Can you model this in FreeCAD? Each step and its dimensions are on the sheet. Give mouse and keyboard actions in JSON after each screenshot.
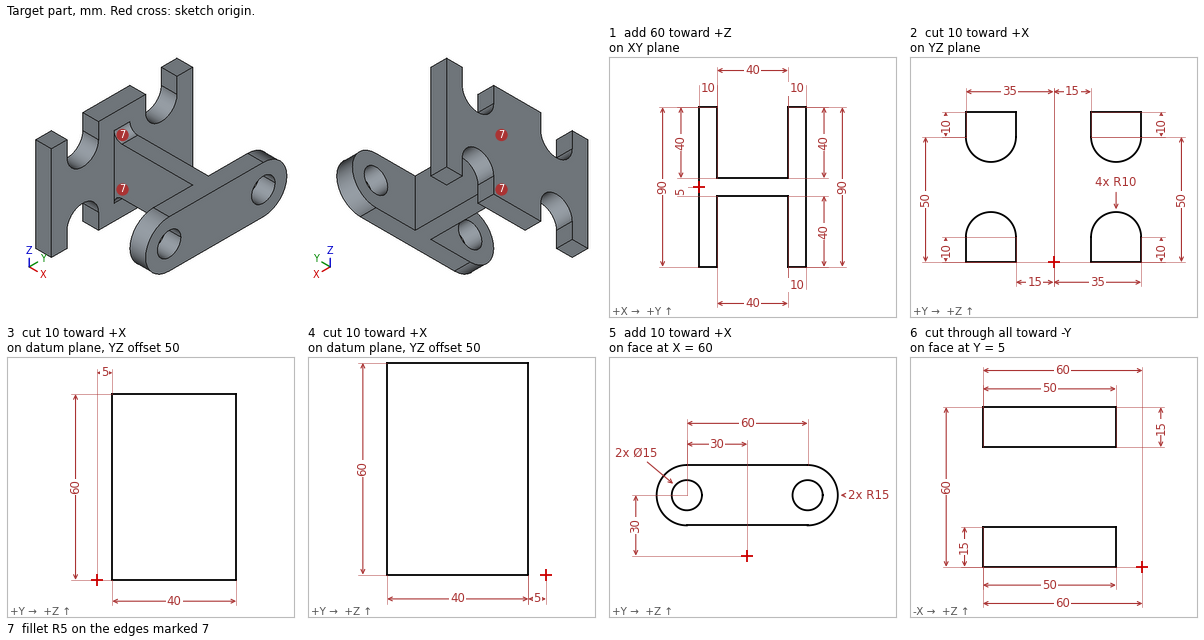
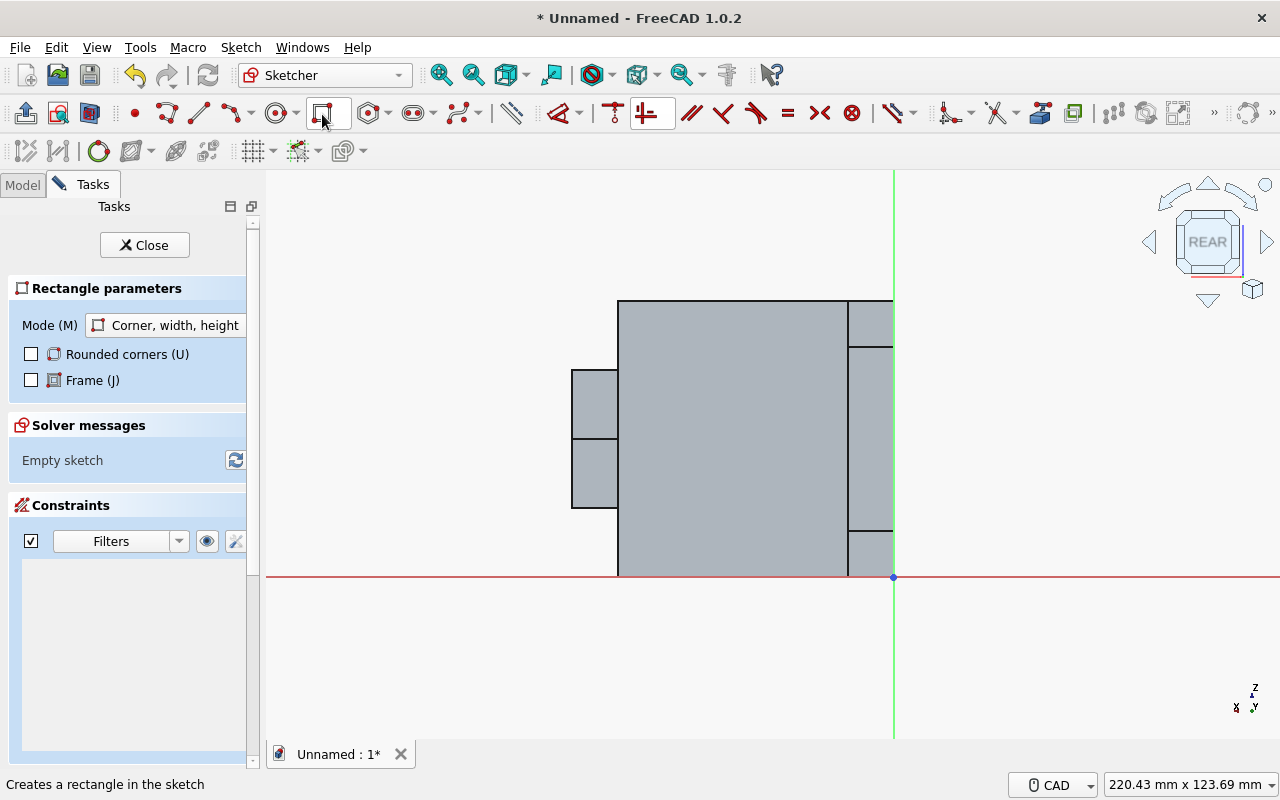
{"action": "left_click", "coordinate": [618, 508]}
{"action": "left_click", "coordinate": [848, 577]}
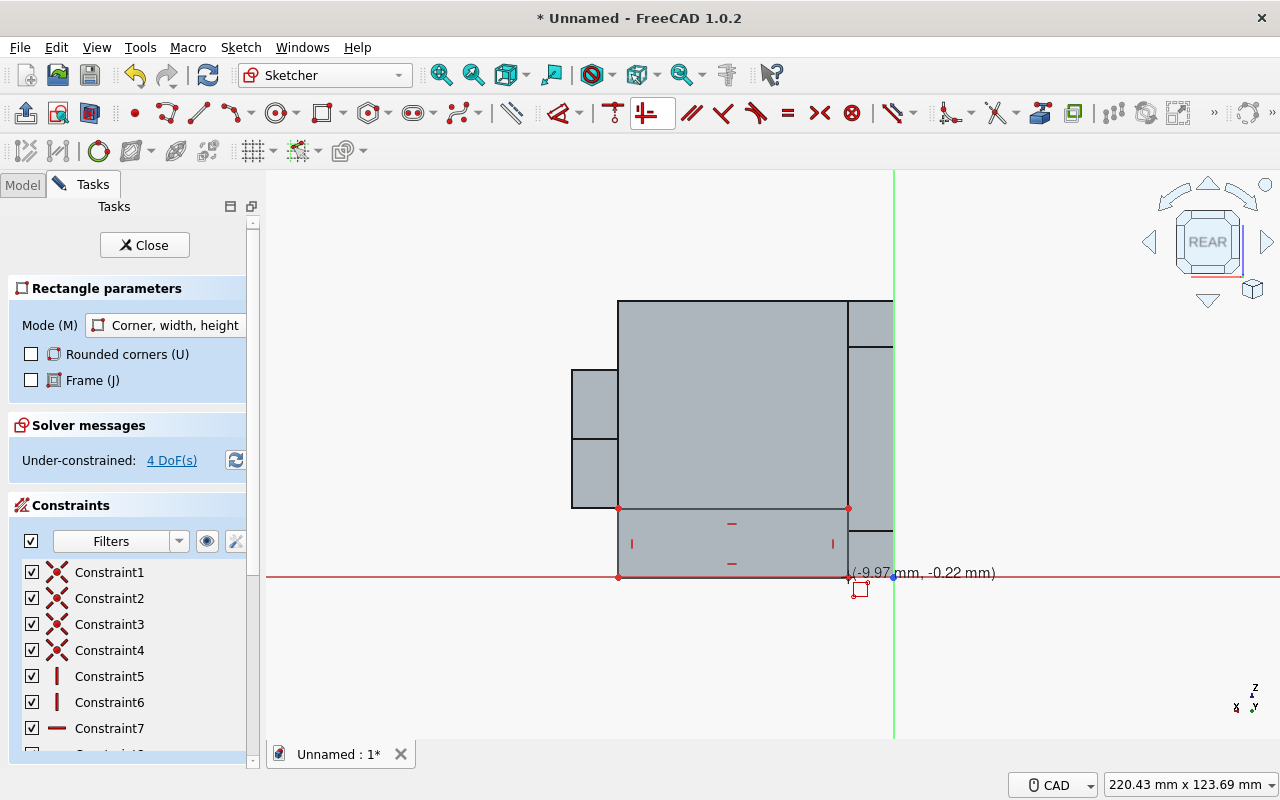
{"action": "left_click", "coordinate": [618, 301]}
{"action": "mouse_move", "coordinate": [848, 370]}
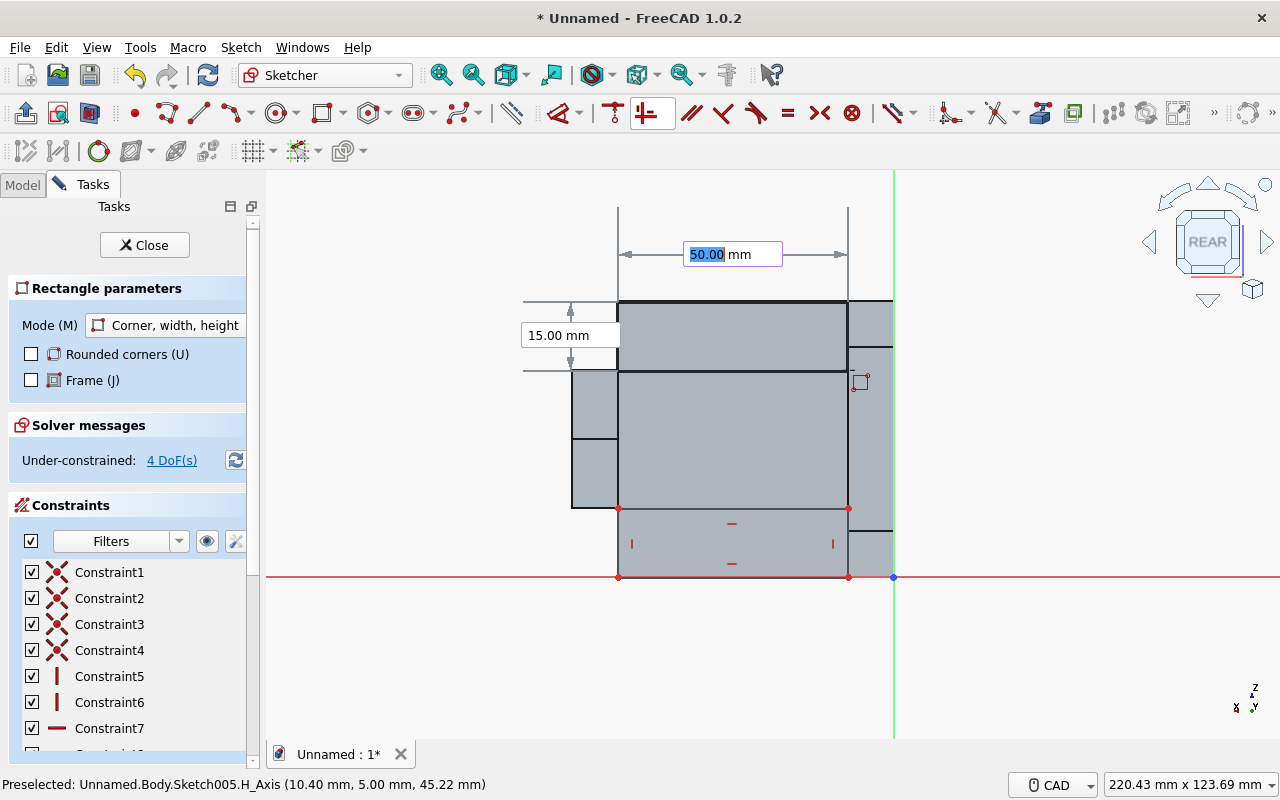
{"action": "type", "text": "50"}
{"action": "key", "text": "Tab"}
{"action": "type", "text": "15"}
{"action": "key", "text": "Return"}
{"action": "key", "text": "Escape"}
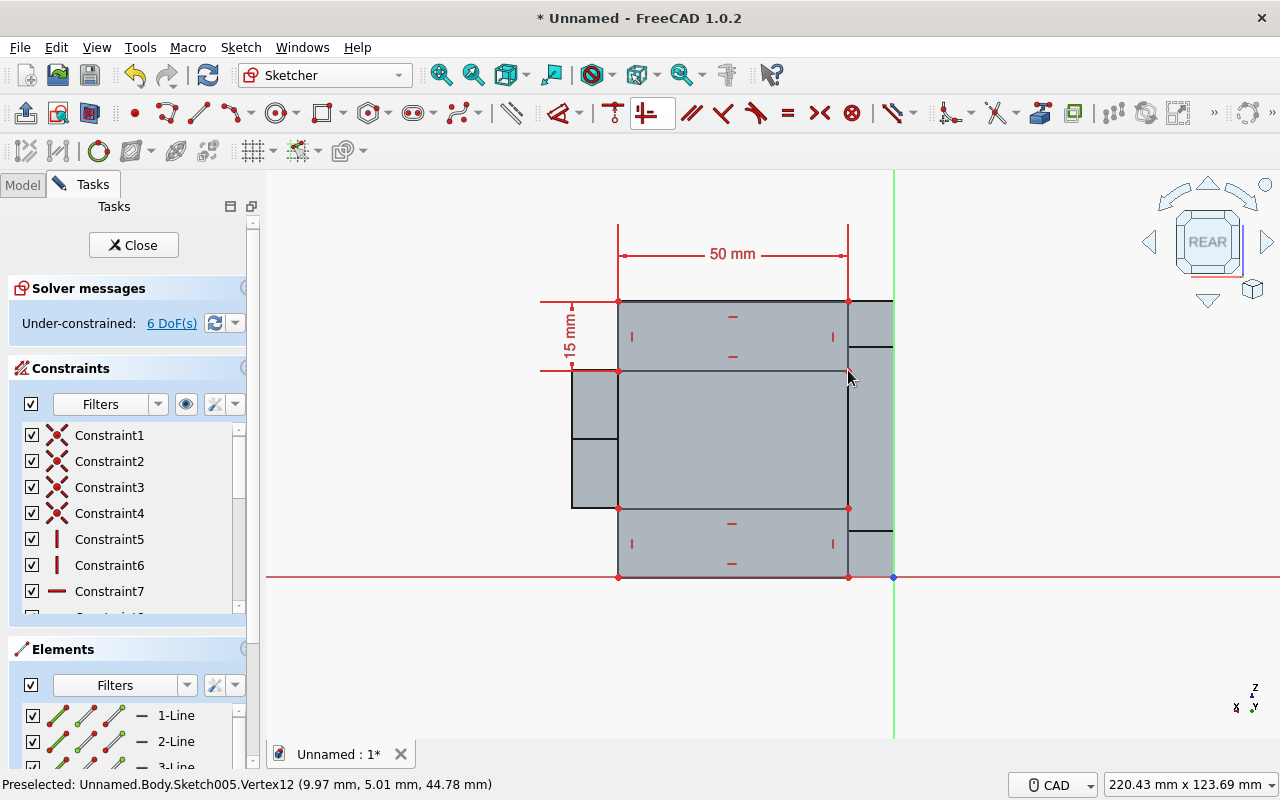
{"action": "left_click", "coordinate": [618, 578]}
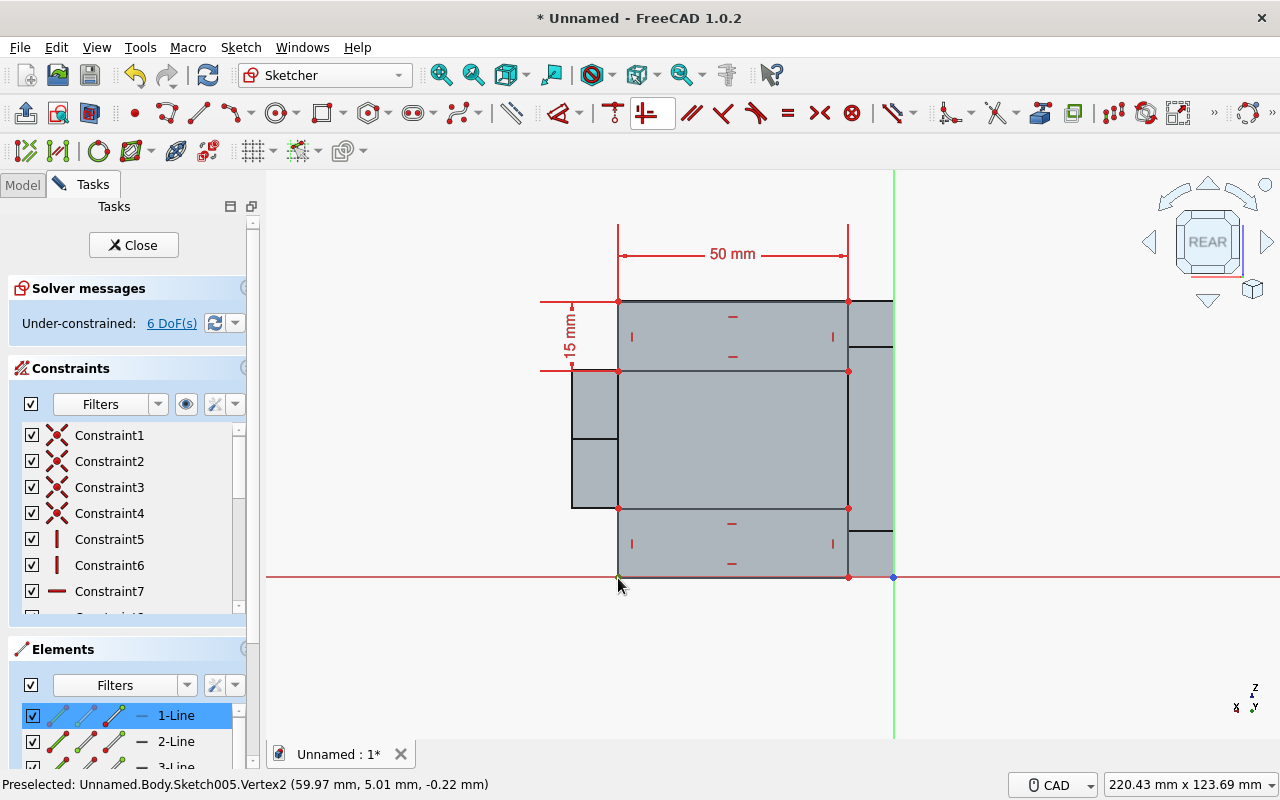
{"action": "left_click", "coordinate": [353, 577]}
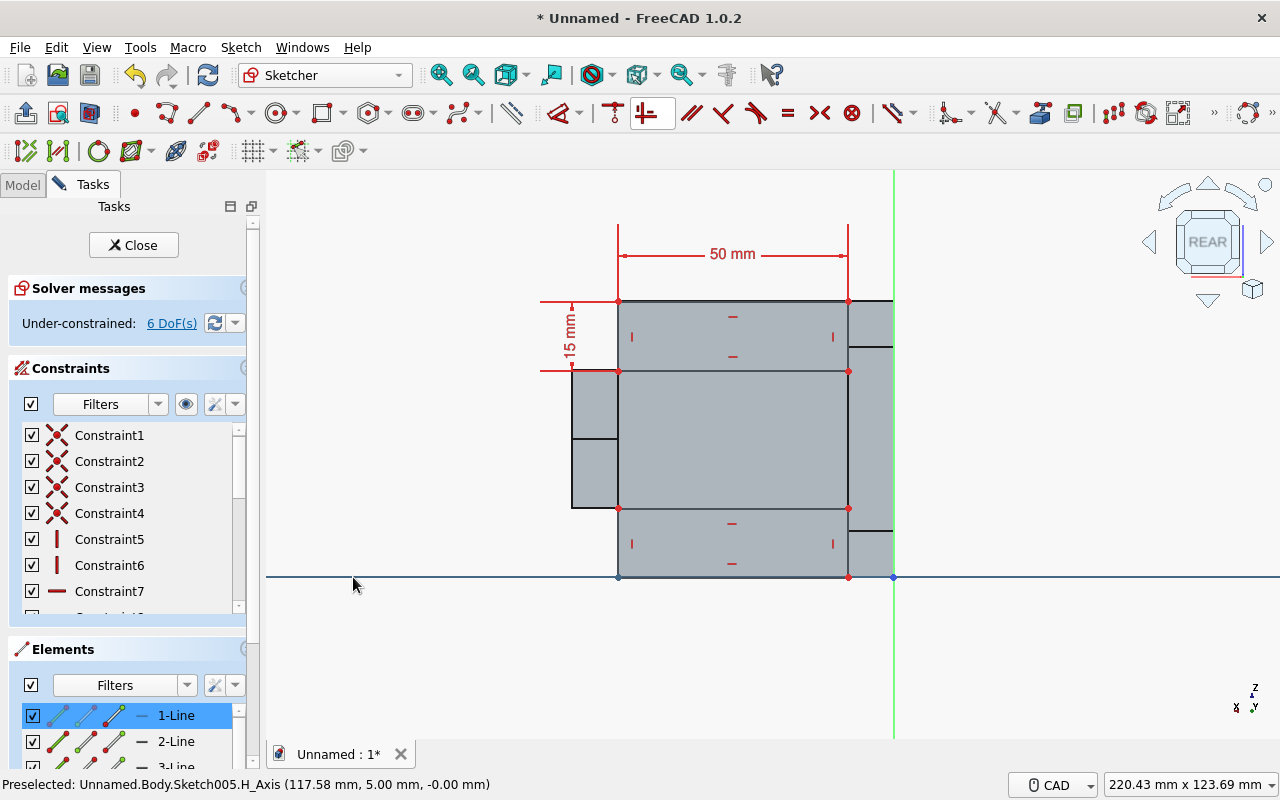
{"action": "left_click", "coordinate": [614, 114]}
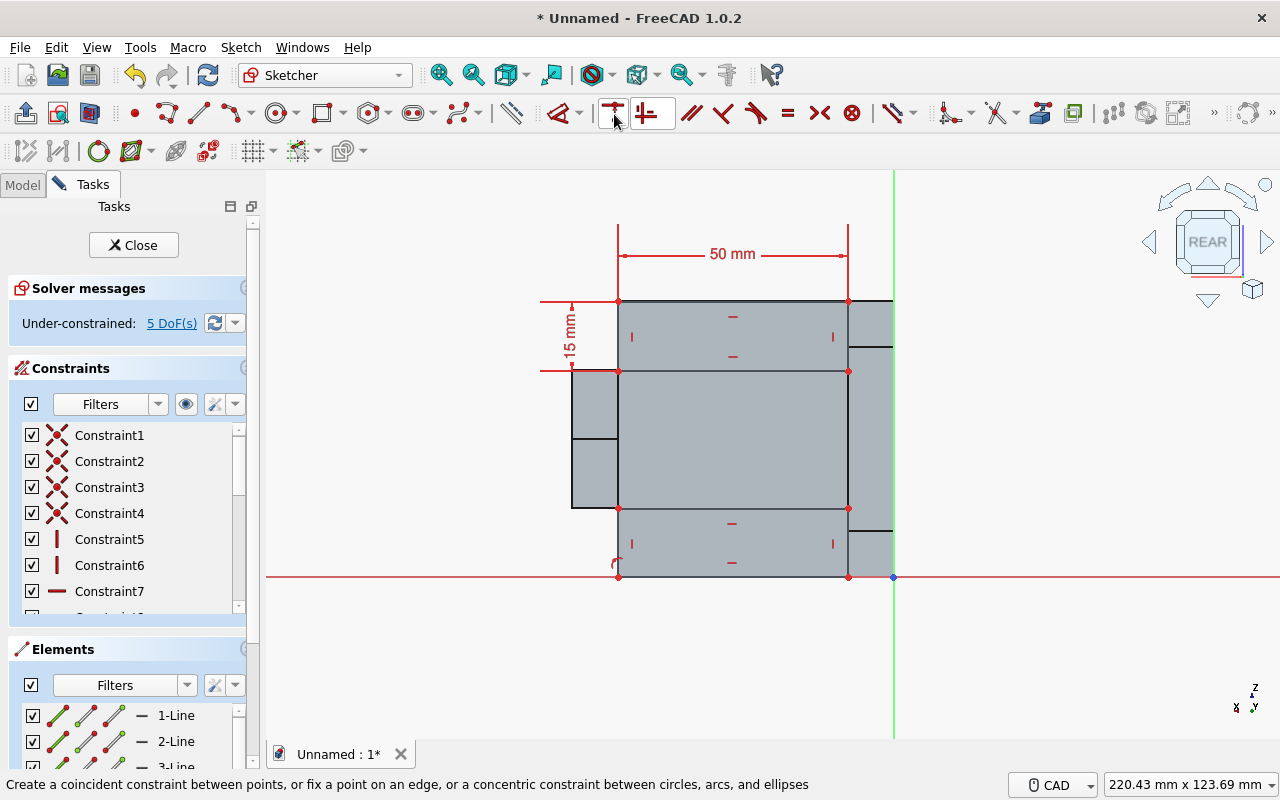
{"action": "left_click", "coordinate": [558, 114]}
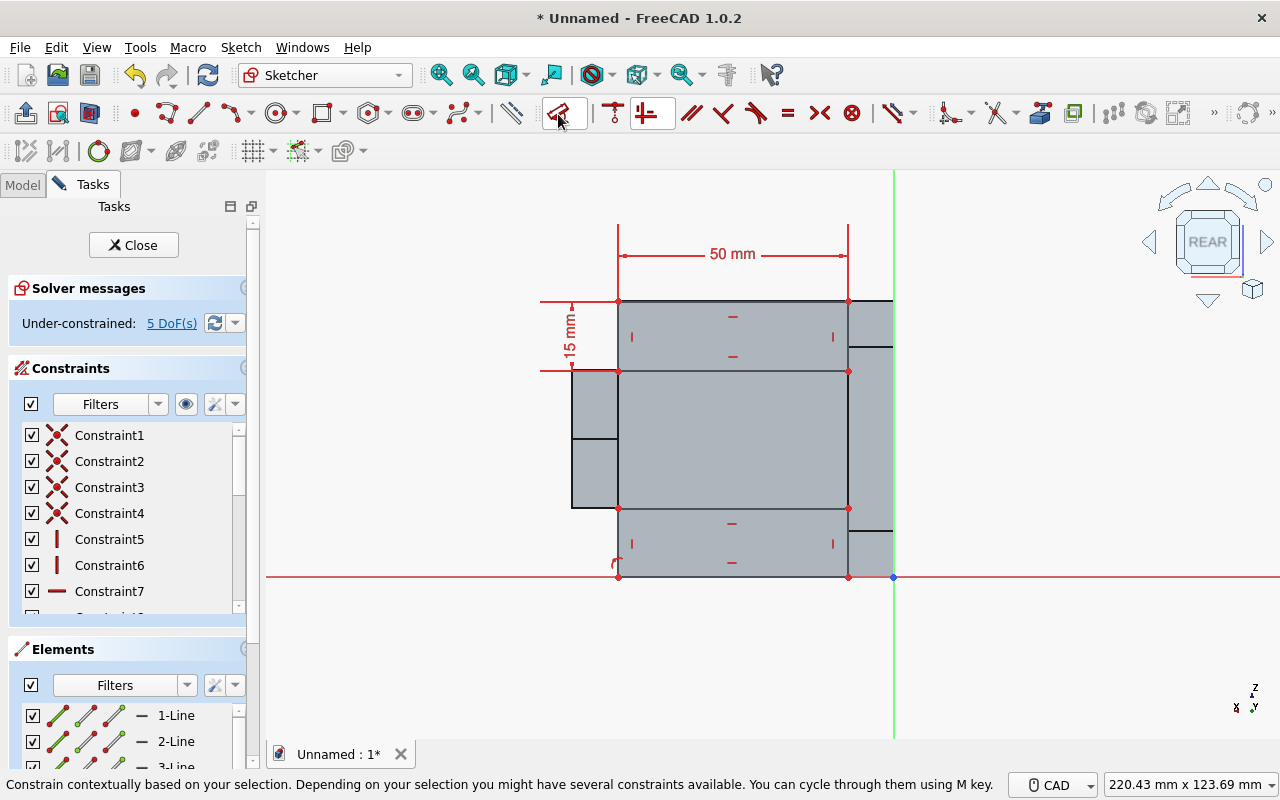
{"action": "left_click", "coordinate": [618, 529]}
{"action": "left_click", "coordinate": [584, 543]}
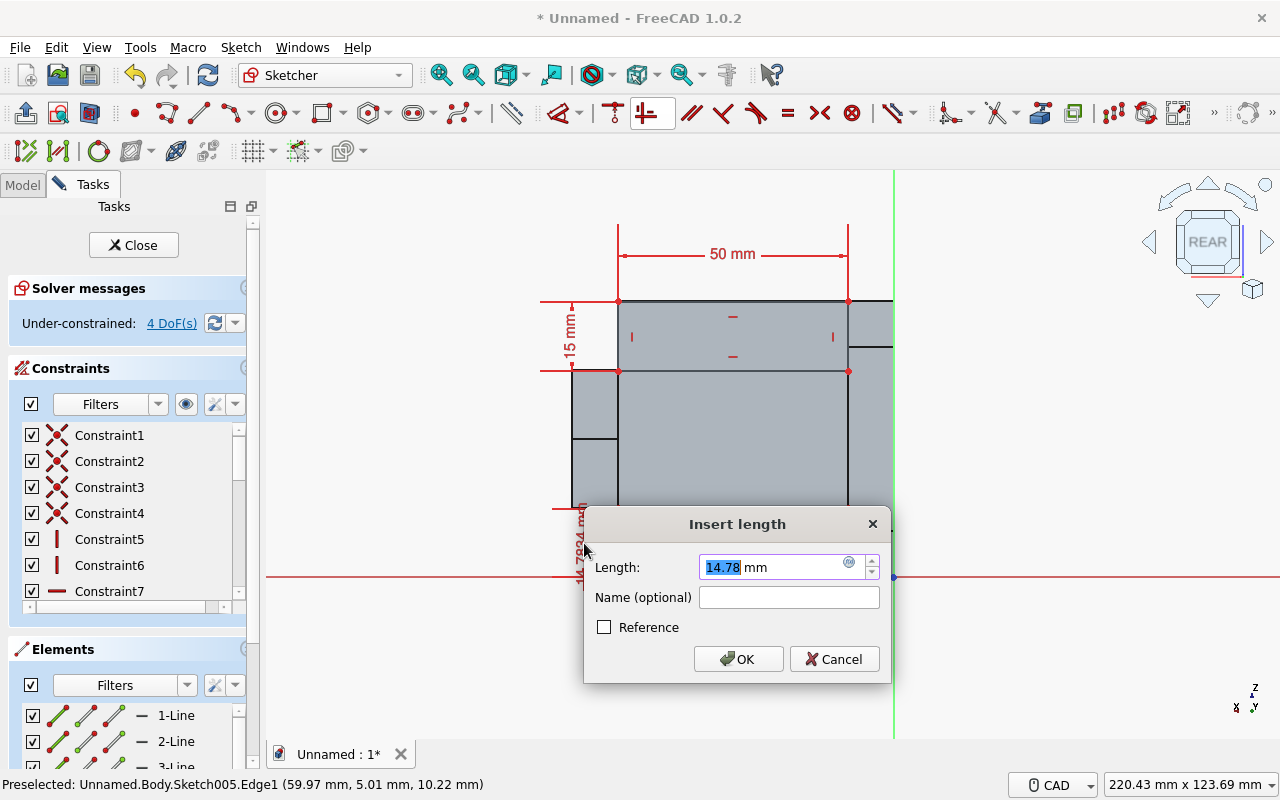
{"action": "type", "text": "15"}
{"action": "key", "text": "Return"}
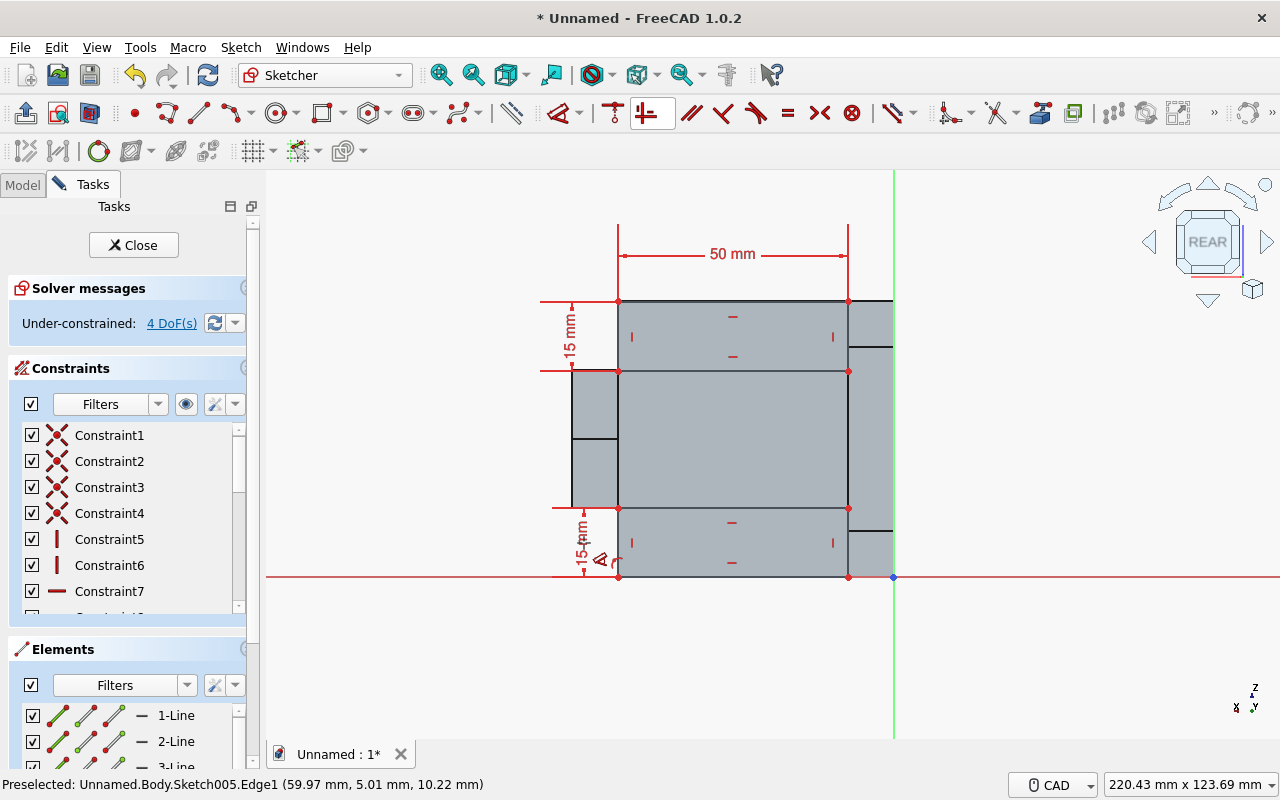
{"action": "left_click", "coordinate": [687, 577]}
{"action": "left_click", "coordinate": [733, 611]}